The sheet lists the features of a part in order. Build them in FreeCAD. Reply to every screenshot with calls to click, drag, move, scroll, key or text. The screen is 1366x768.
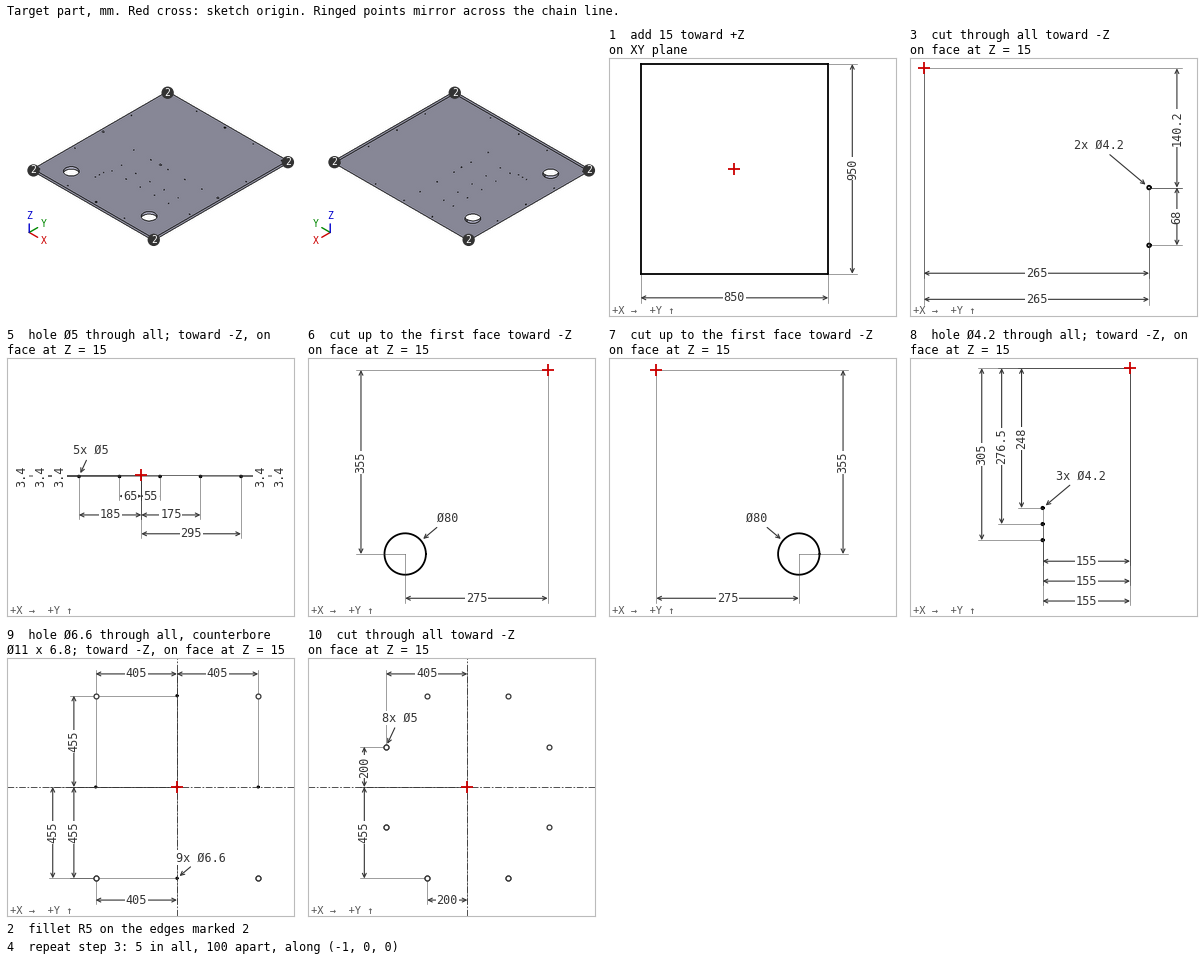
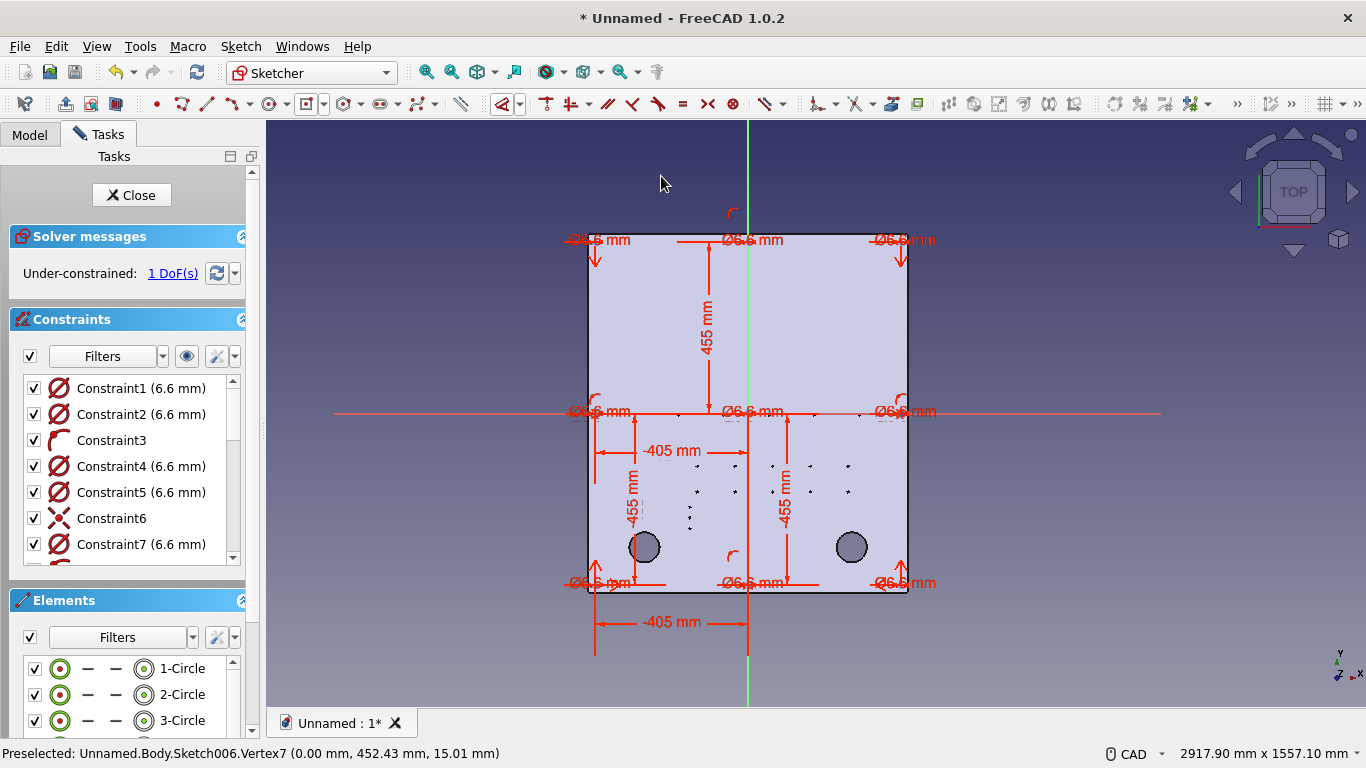
click(901, 414)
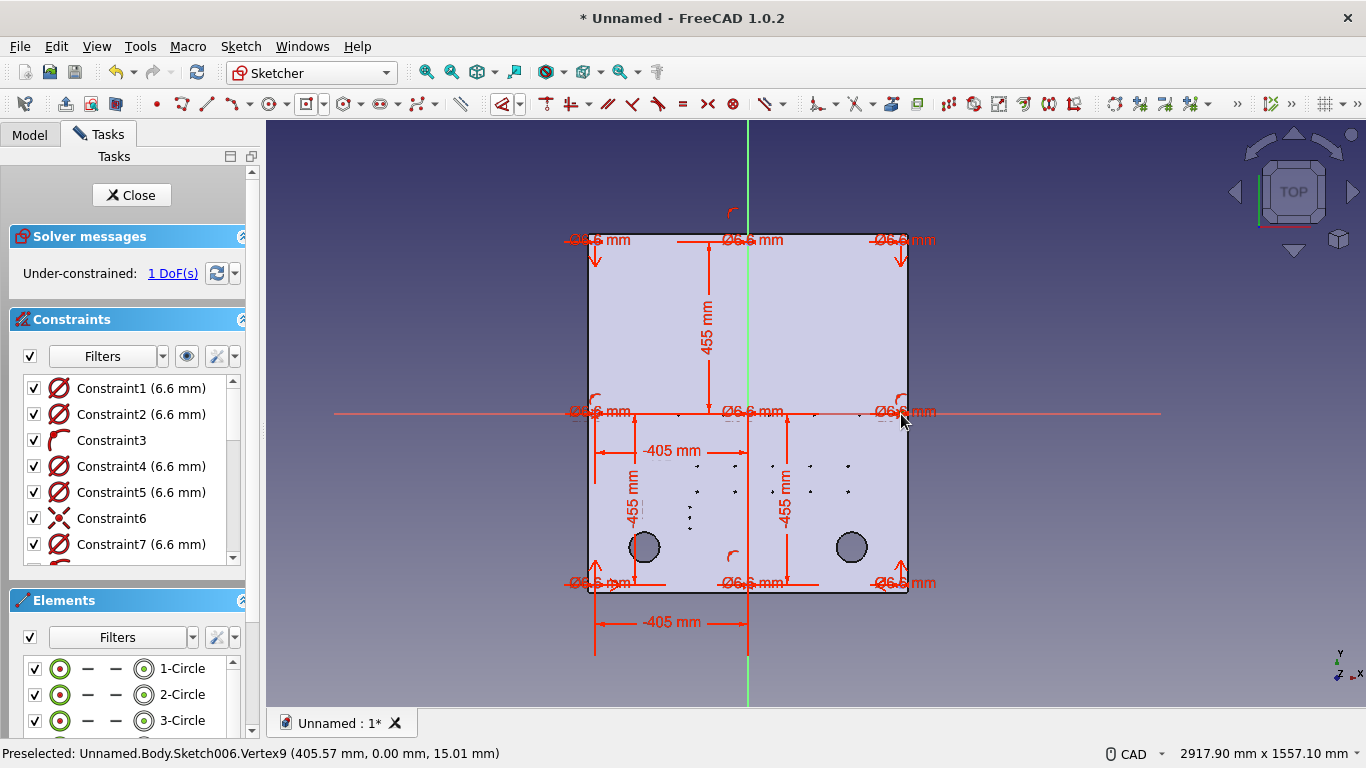
key(l)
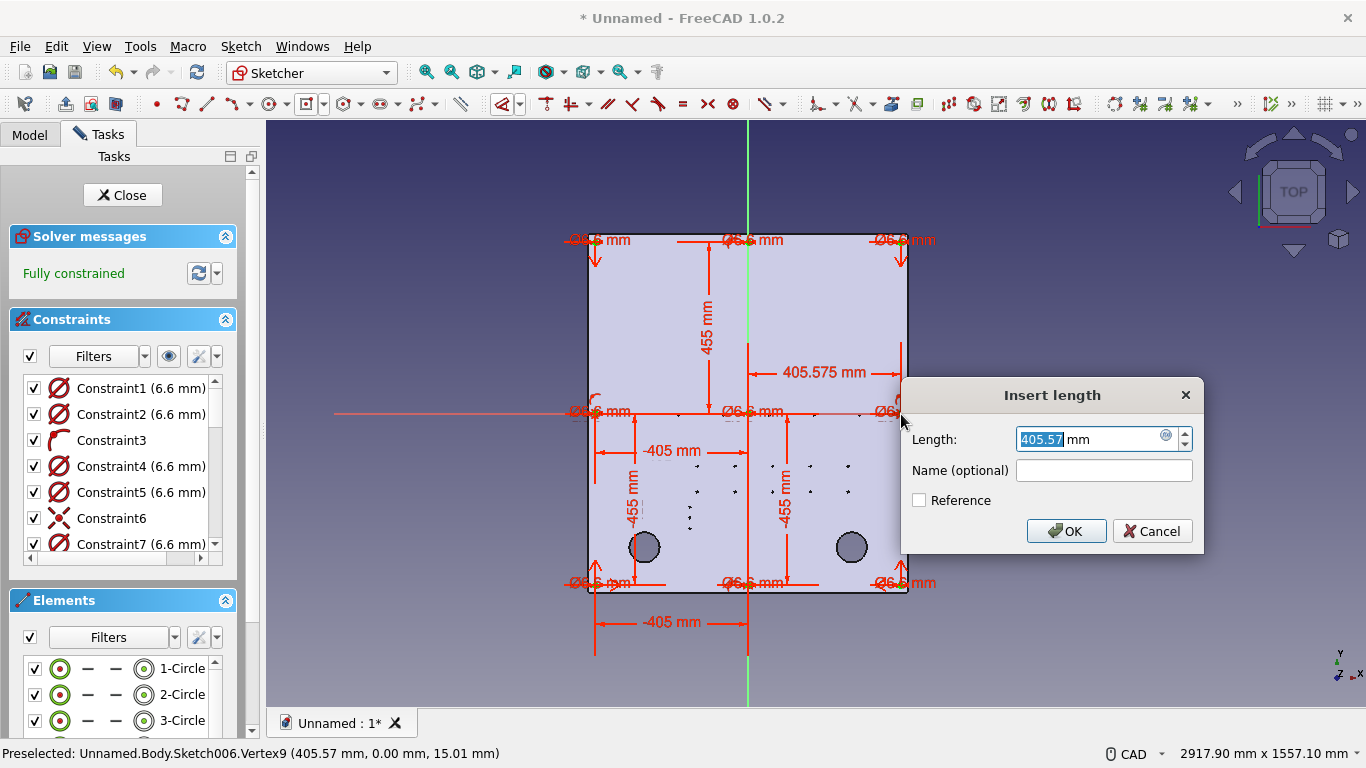
text(405)
key(Return)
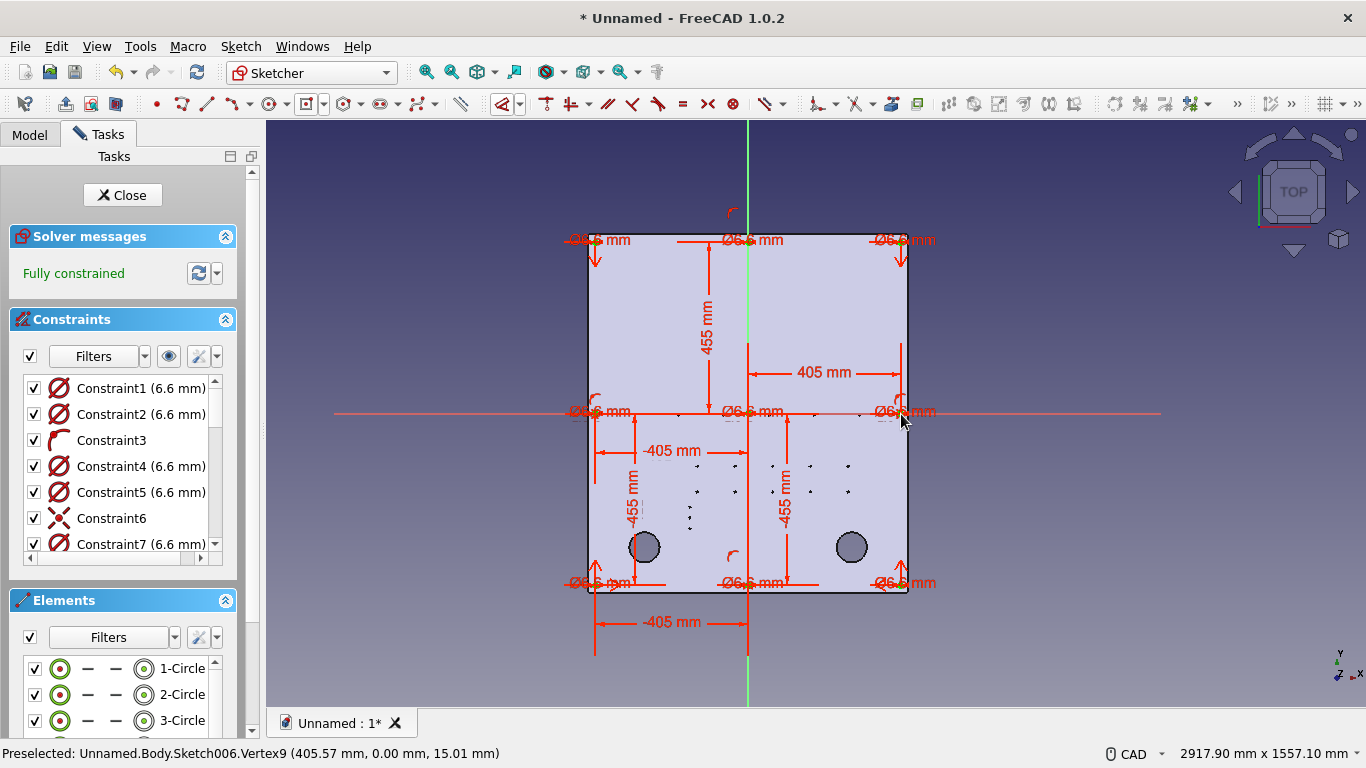
click(123, 195)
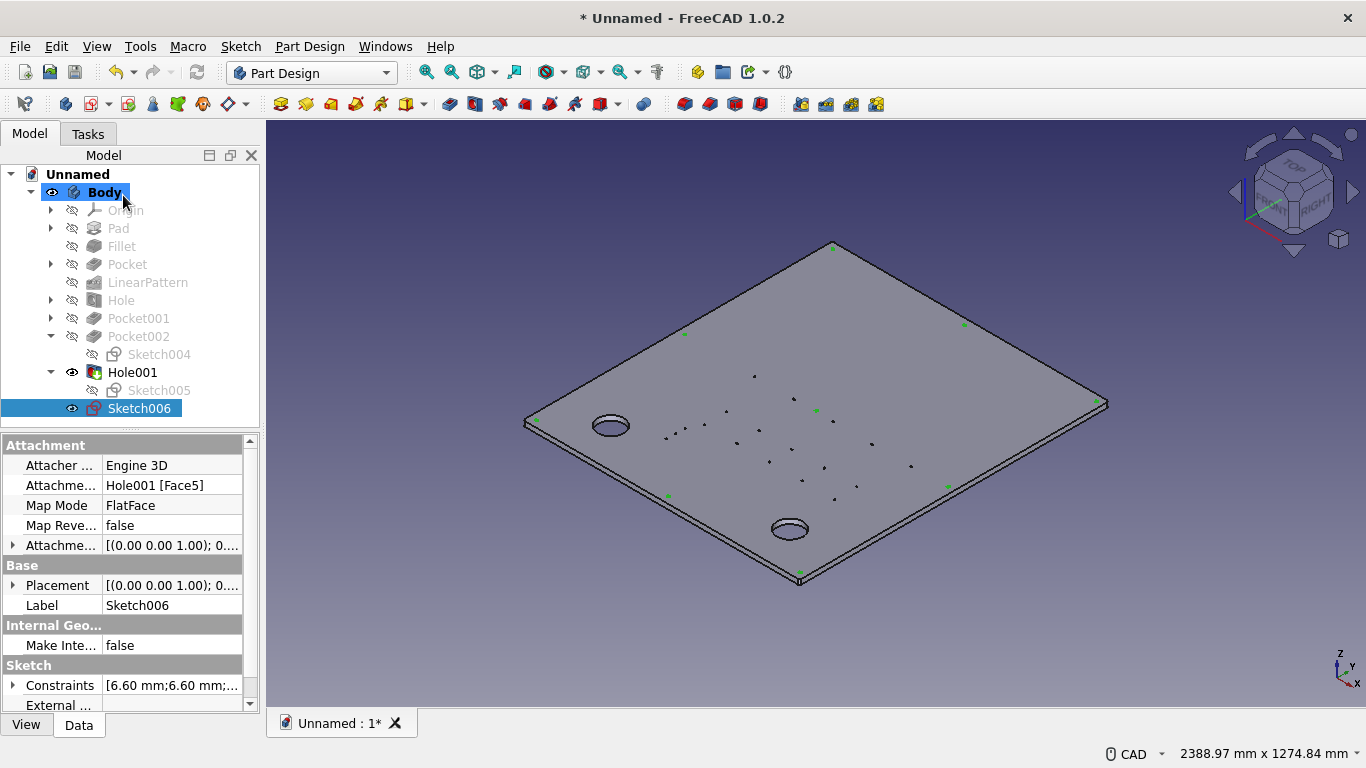
click(475, 104)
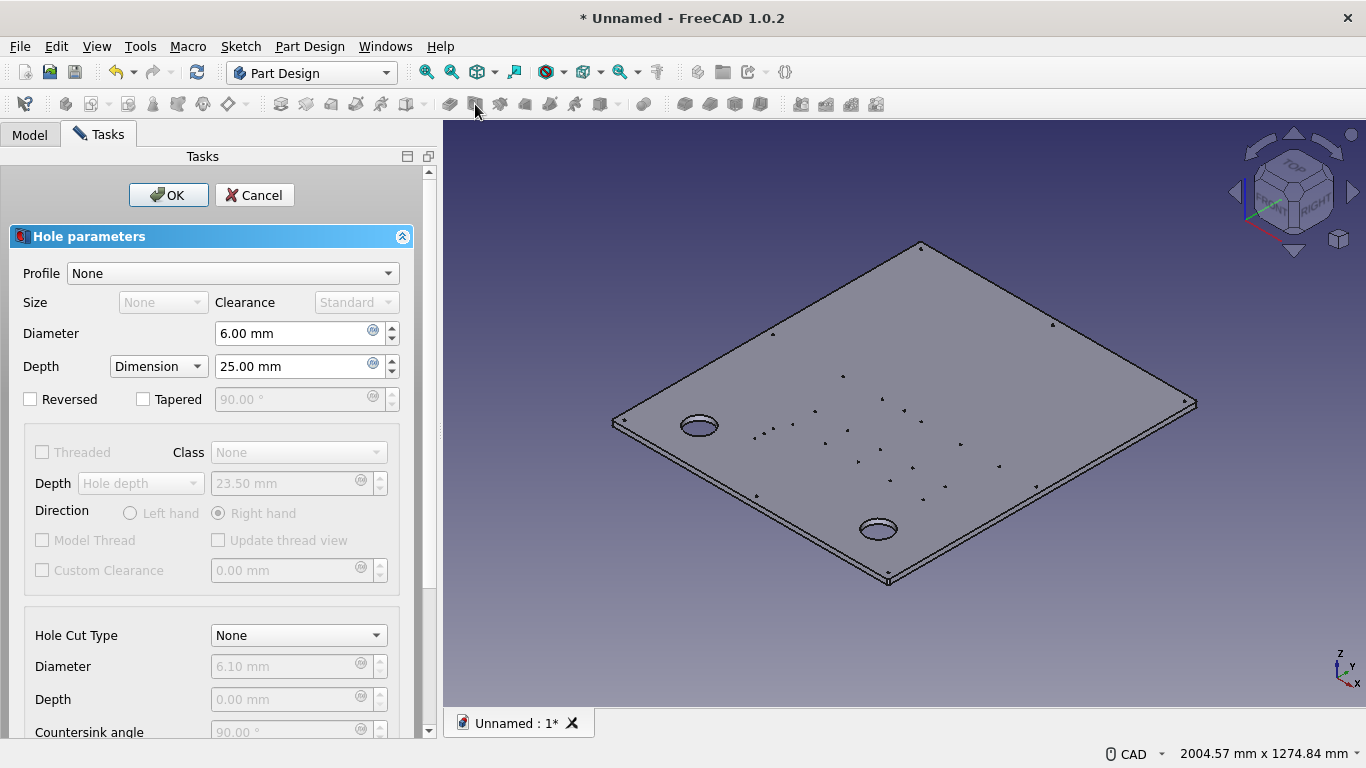
triple_click(300, 334)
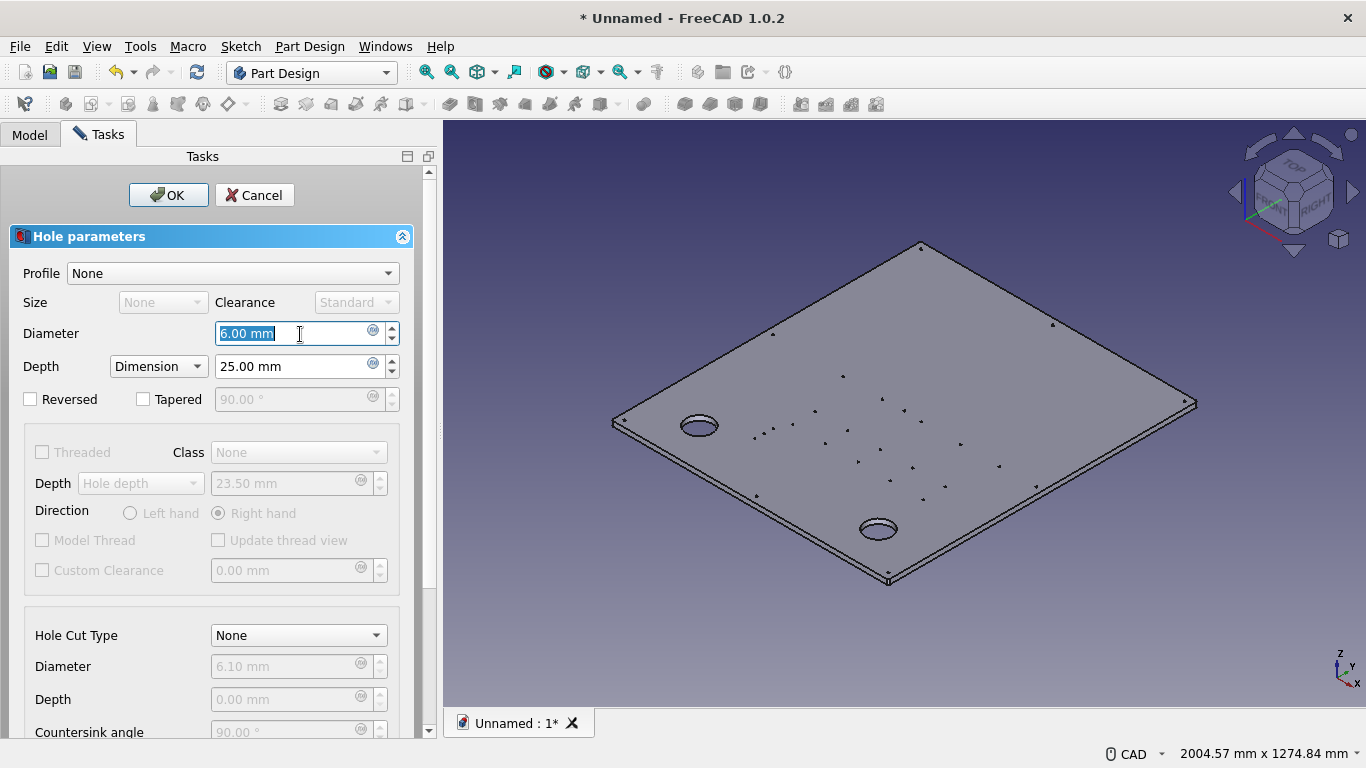
text(6.6)
key(Tab)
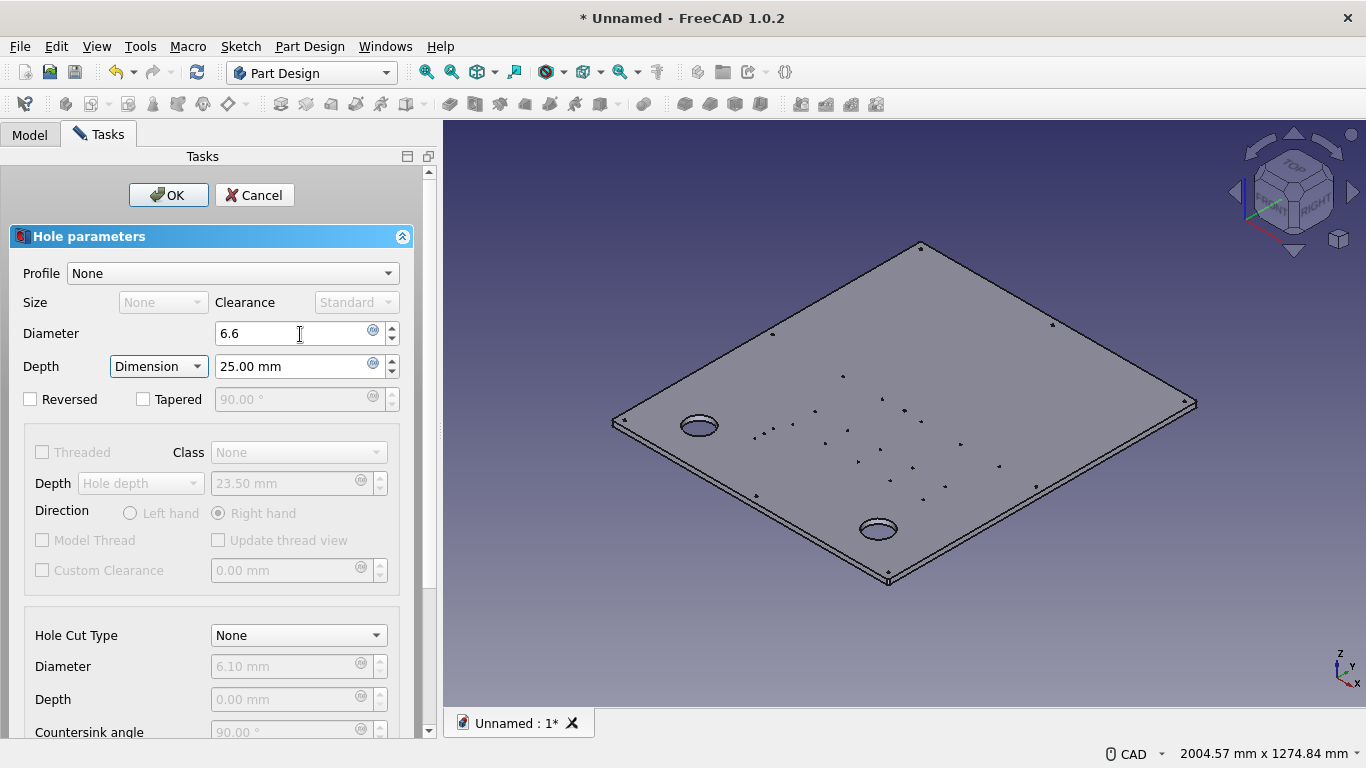
click(160, 366)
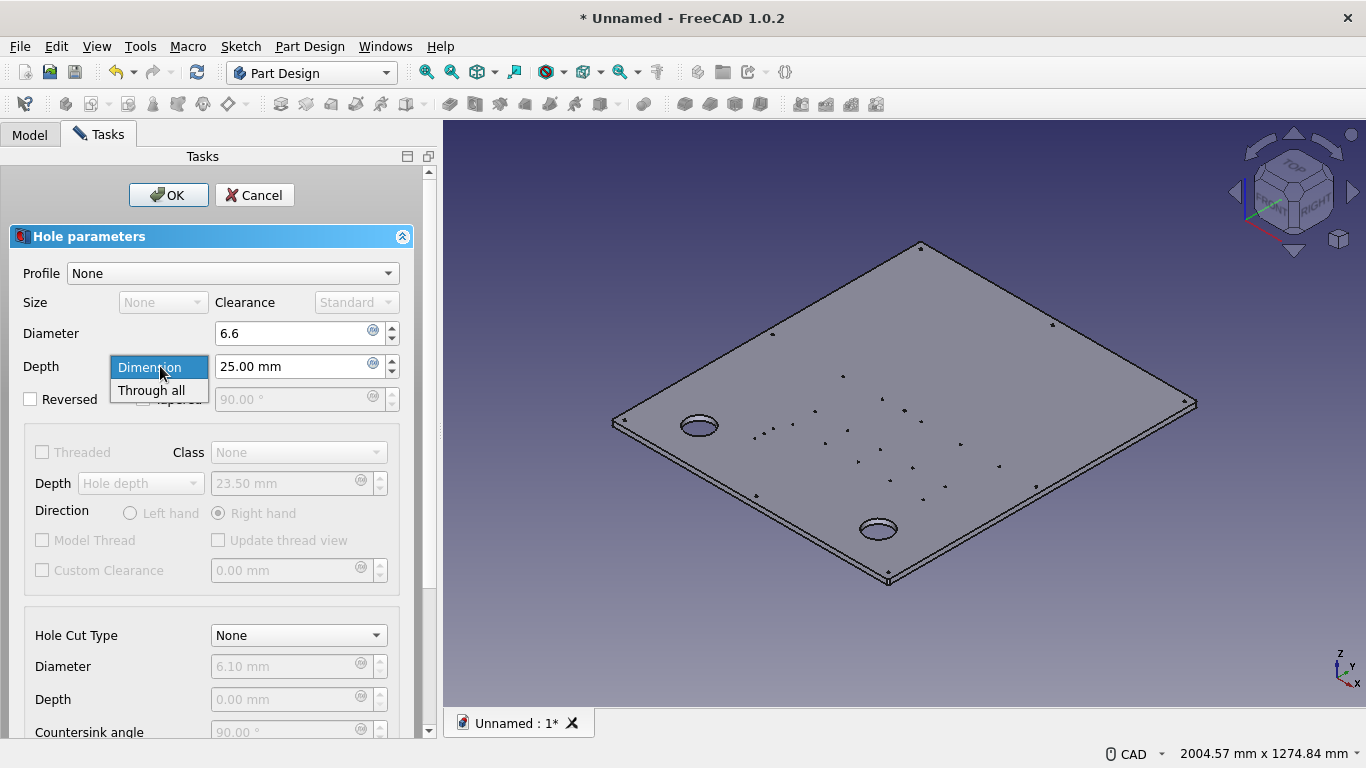
click(158, 390)